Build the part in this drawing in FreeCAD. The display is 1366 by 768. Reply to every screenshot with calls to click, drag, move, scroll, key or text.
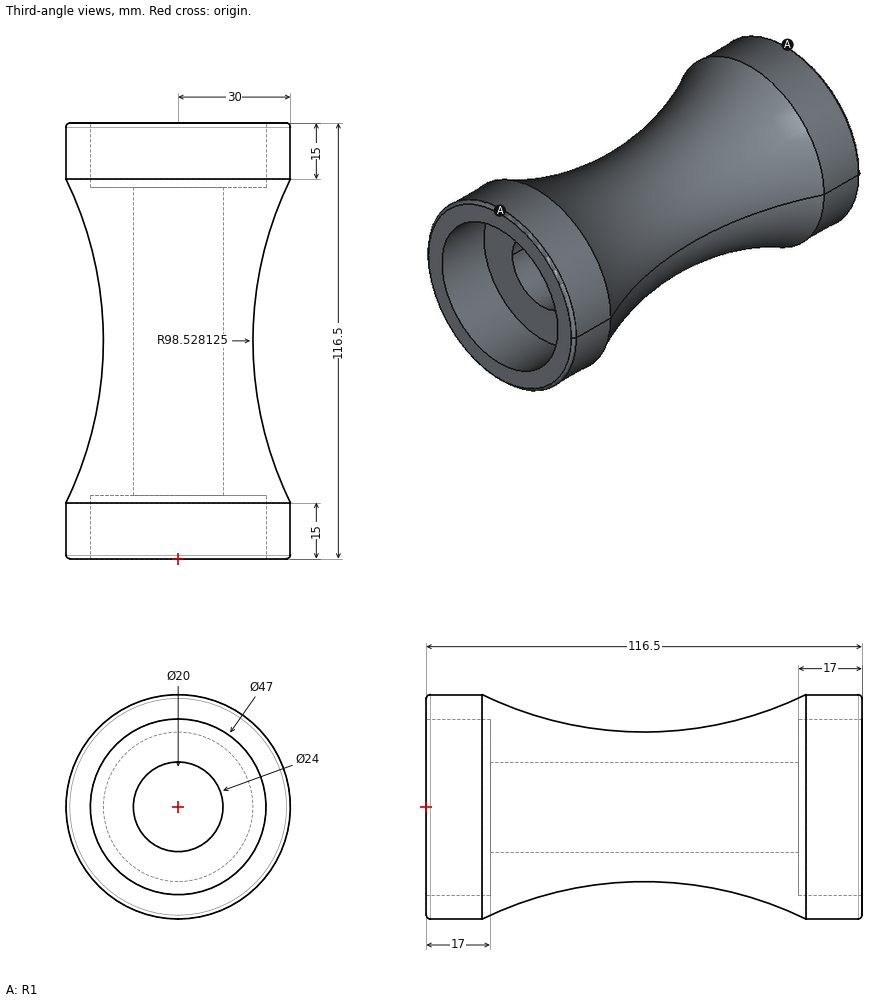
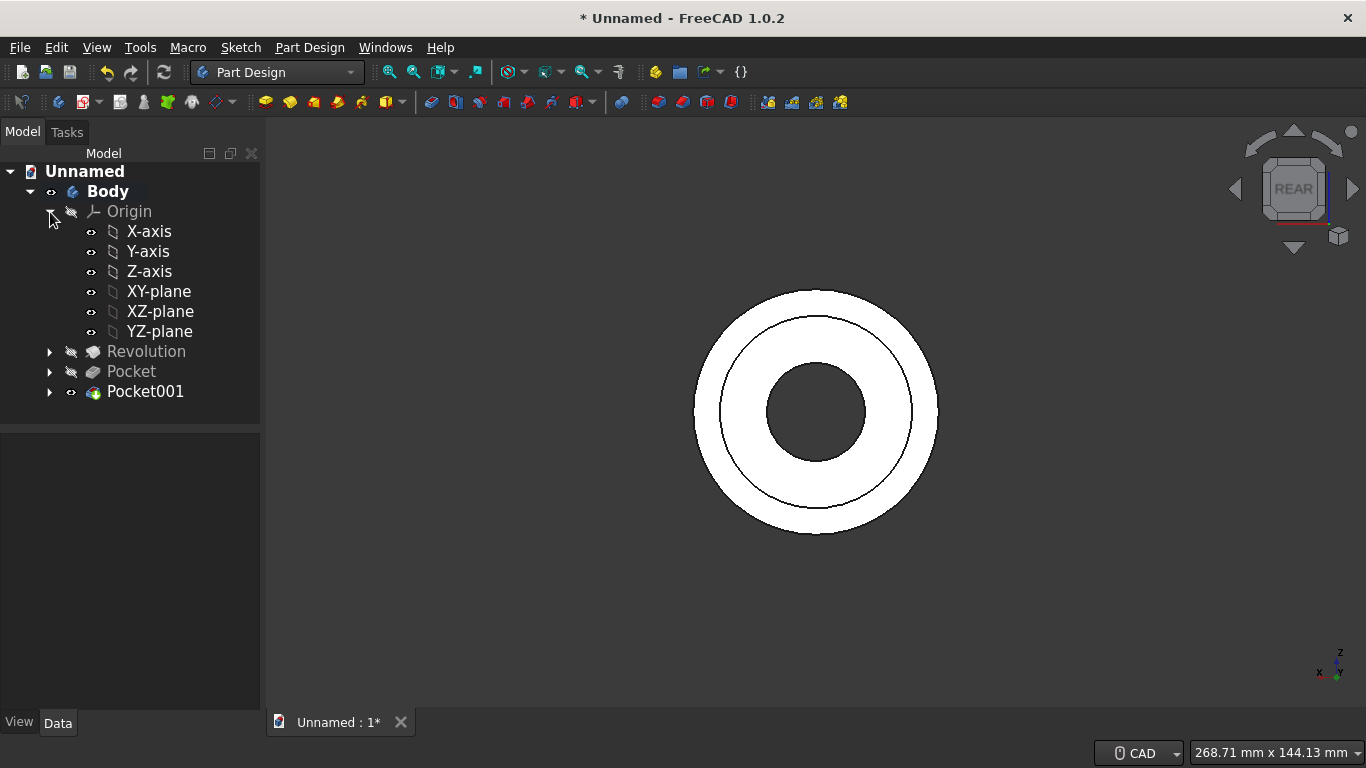
click(136, 312)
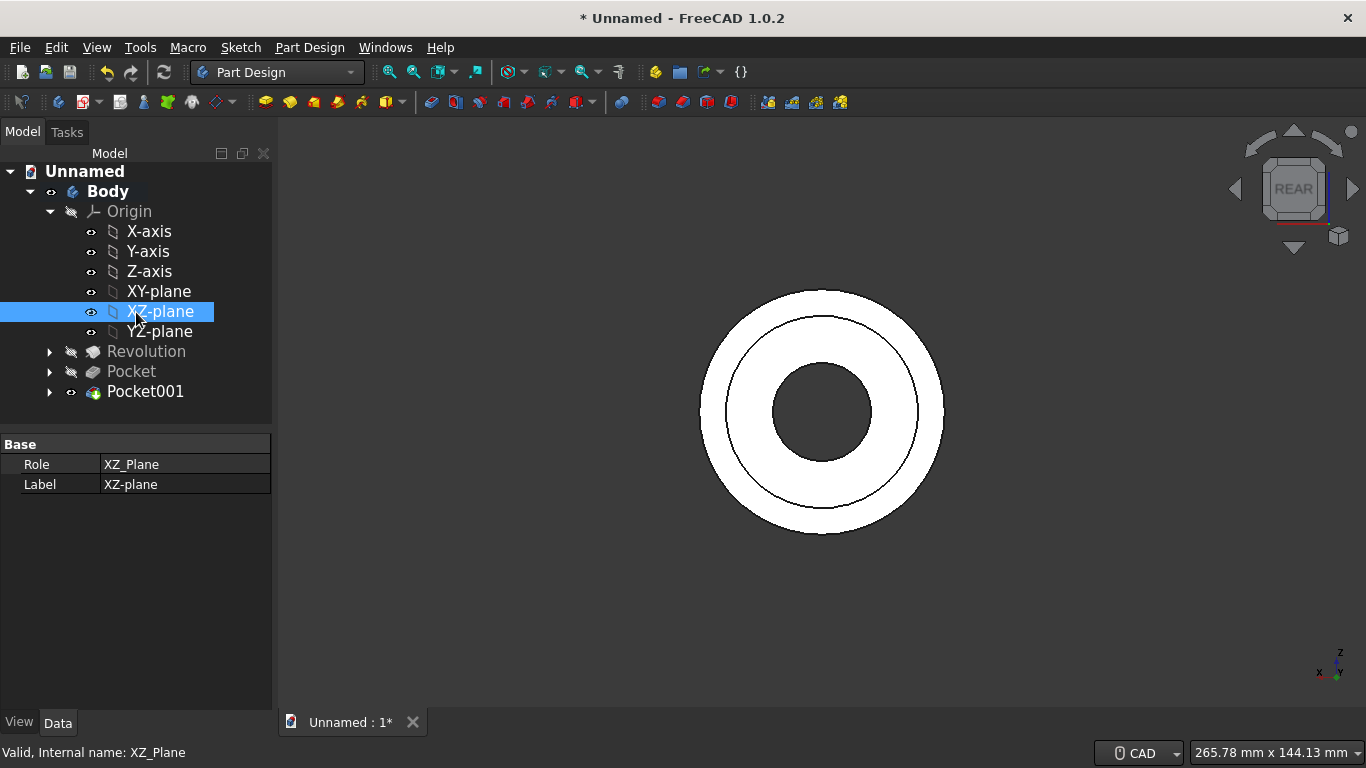
click(216, 102)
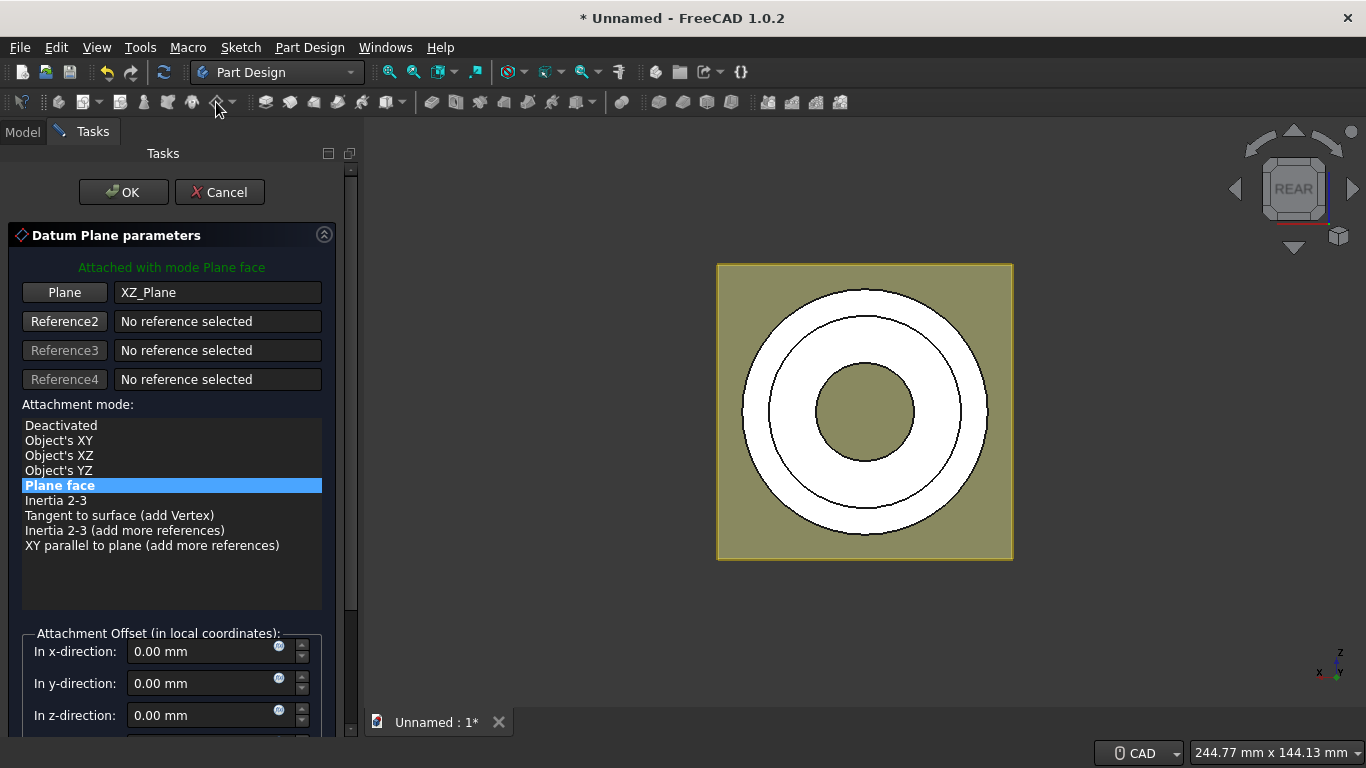
triple_click(210, 715)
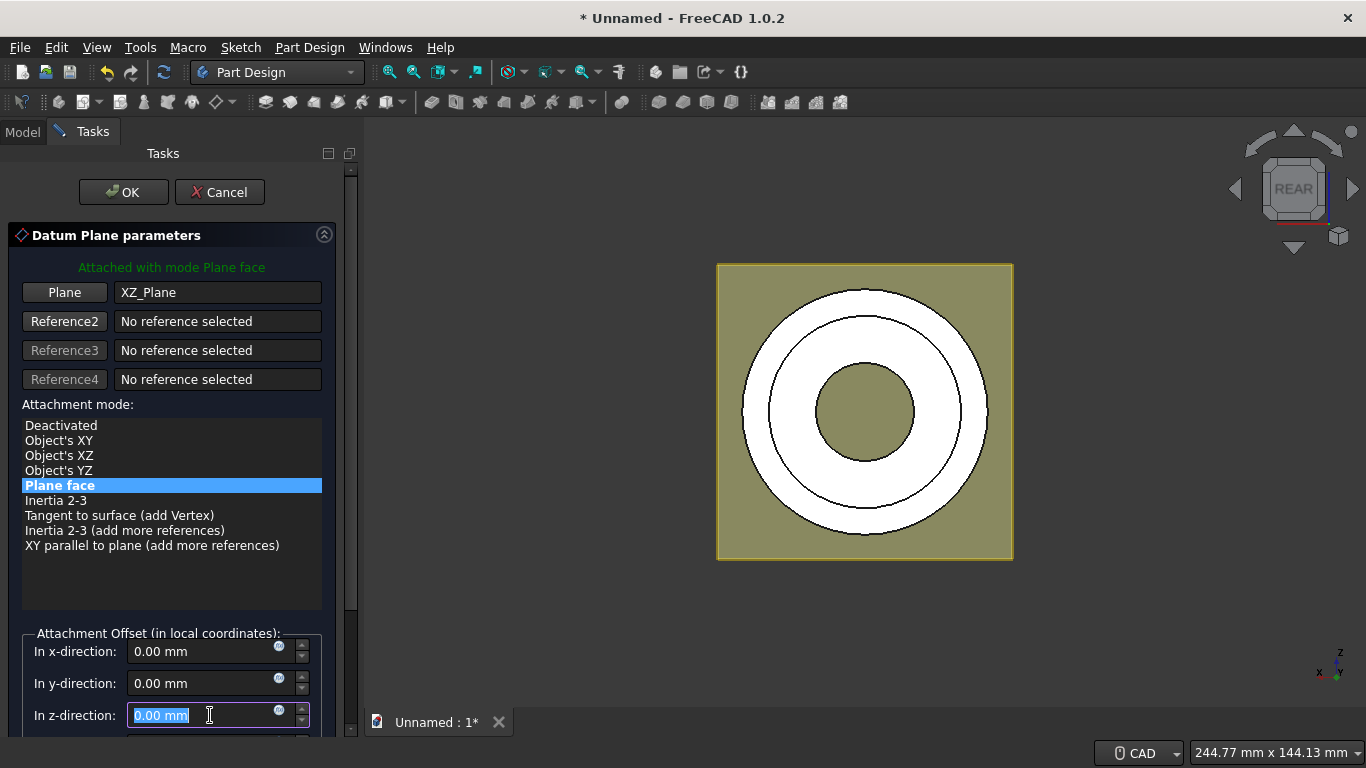
text(-17)
key(Tab)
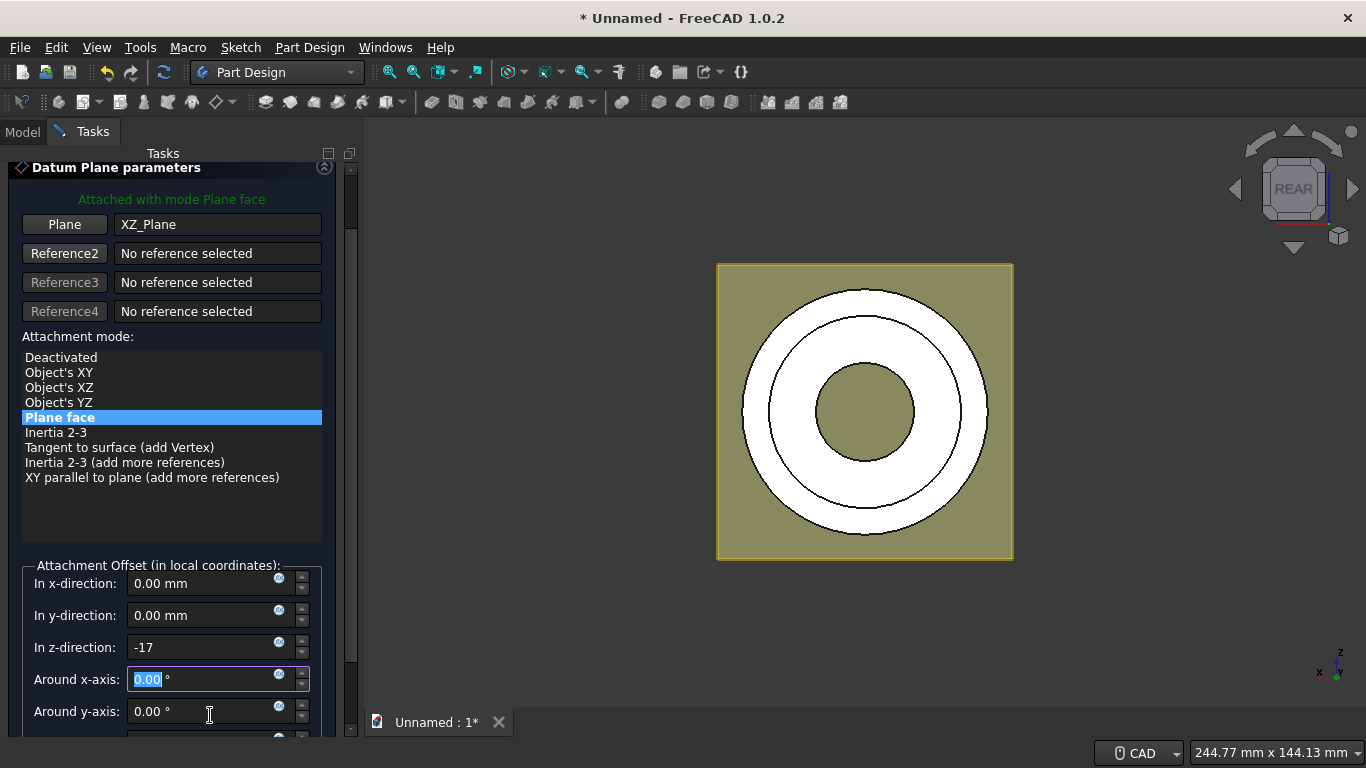
scroll(351, 450, up, 2)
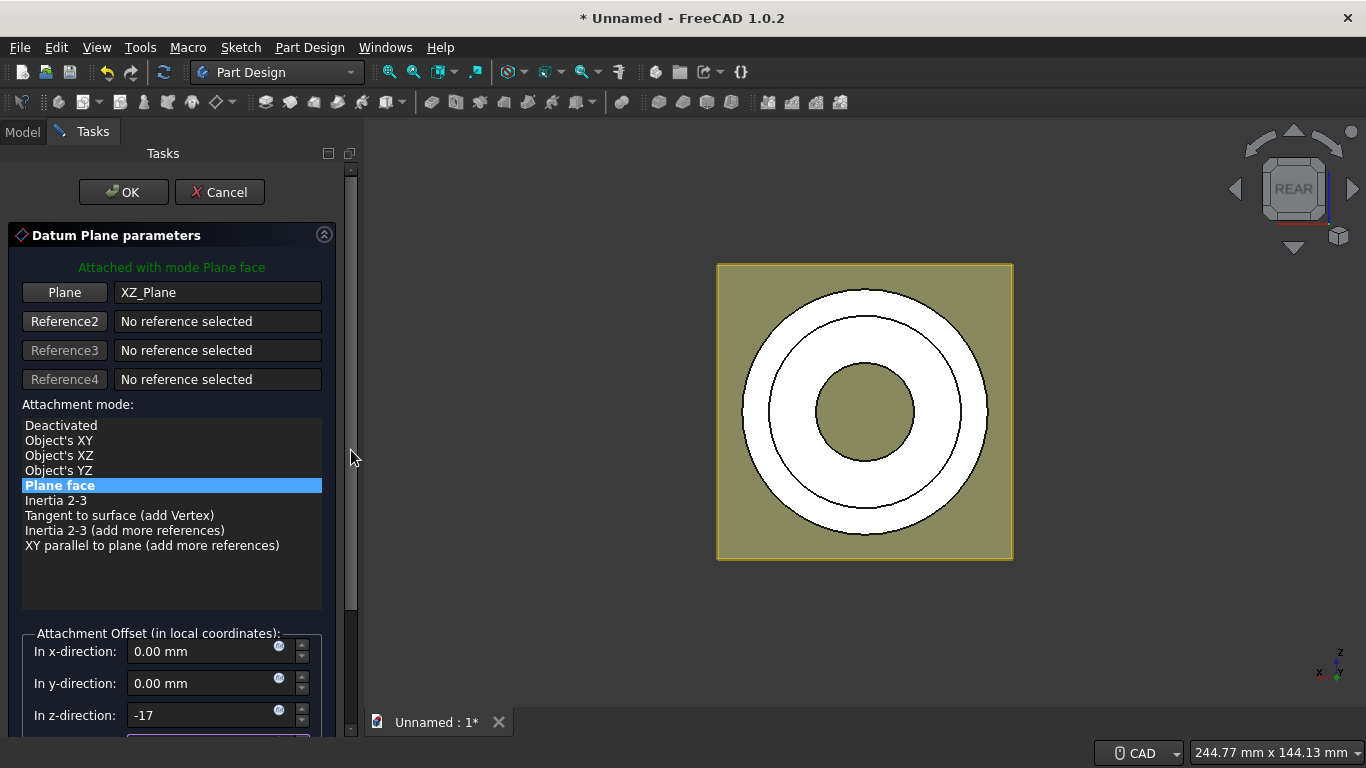
click(124, 192)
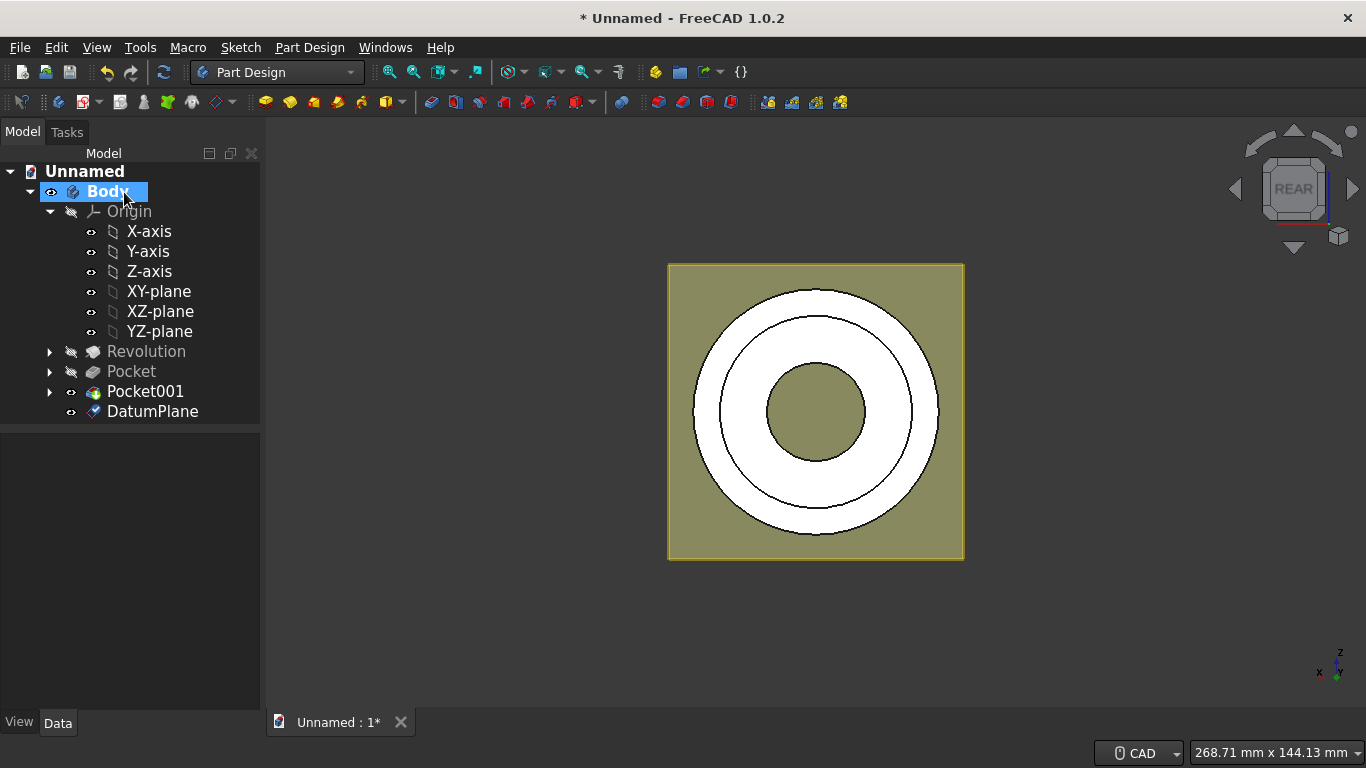
click(116, 412)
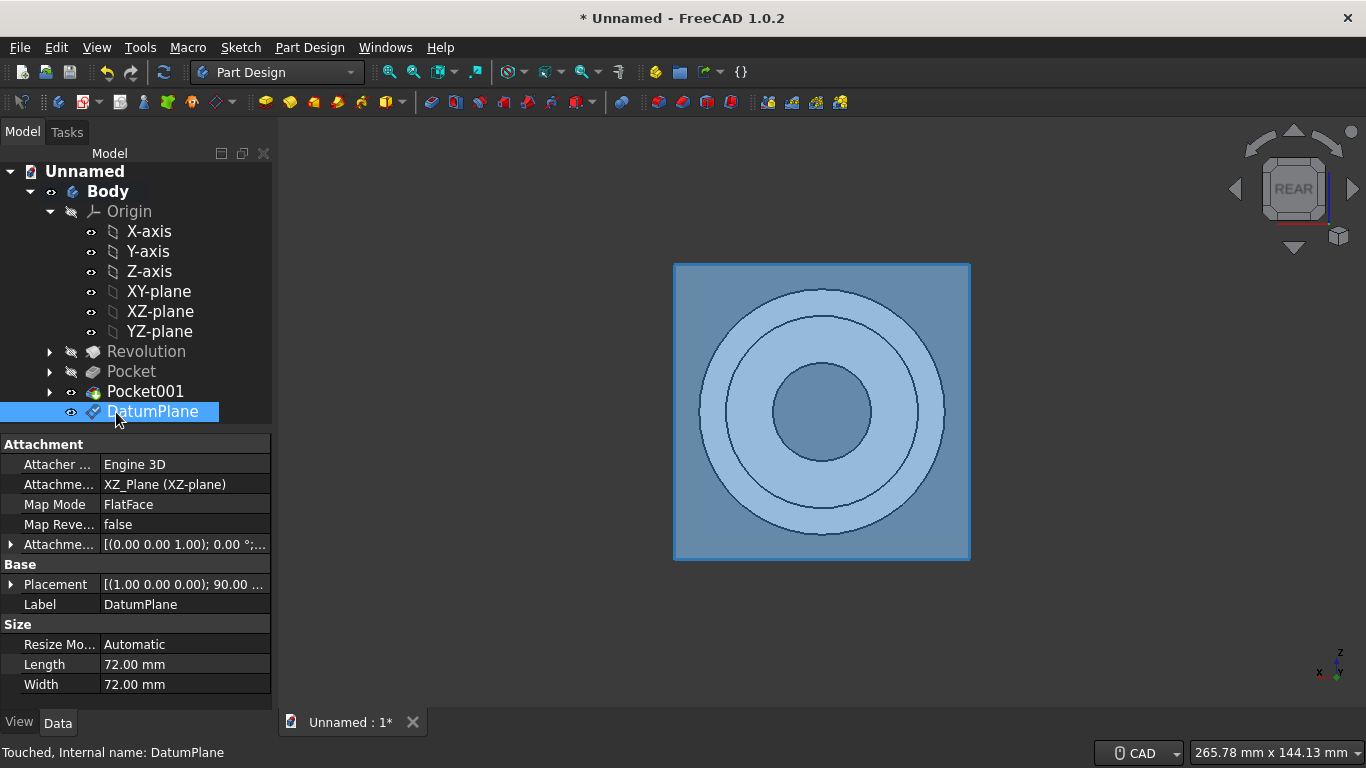
click(84, 102)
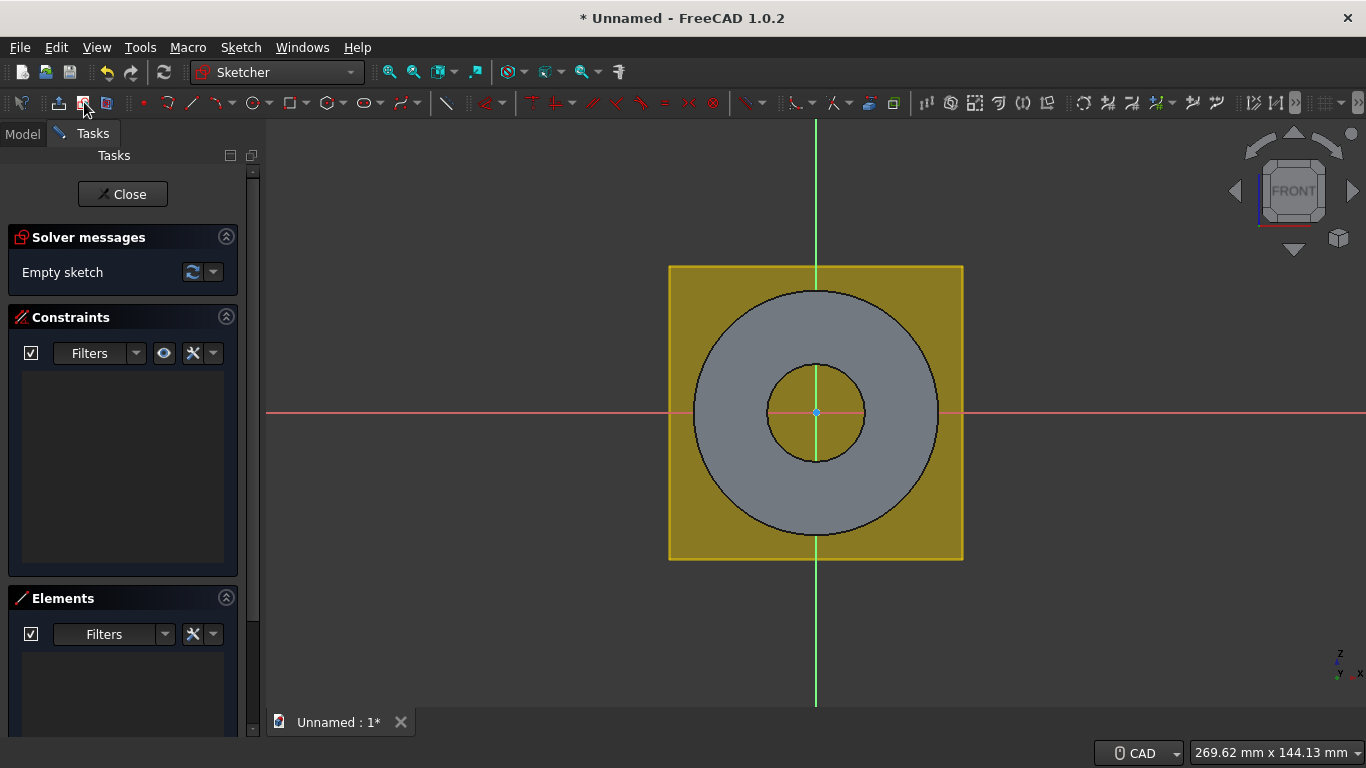
click(108, 104)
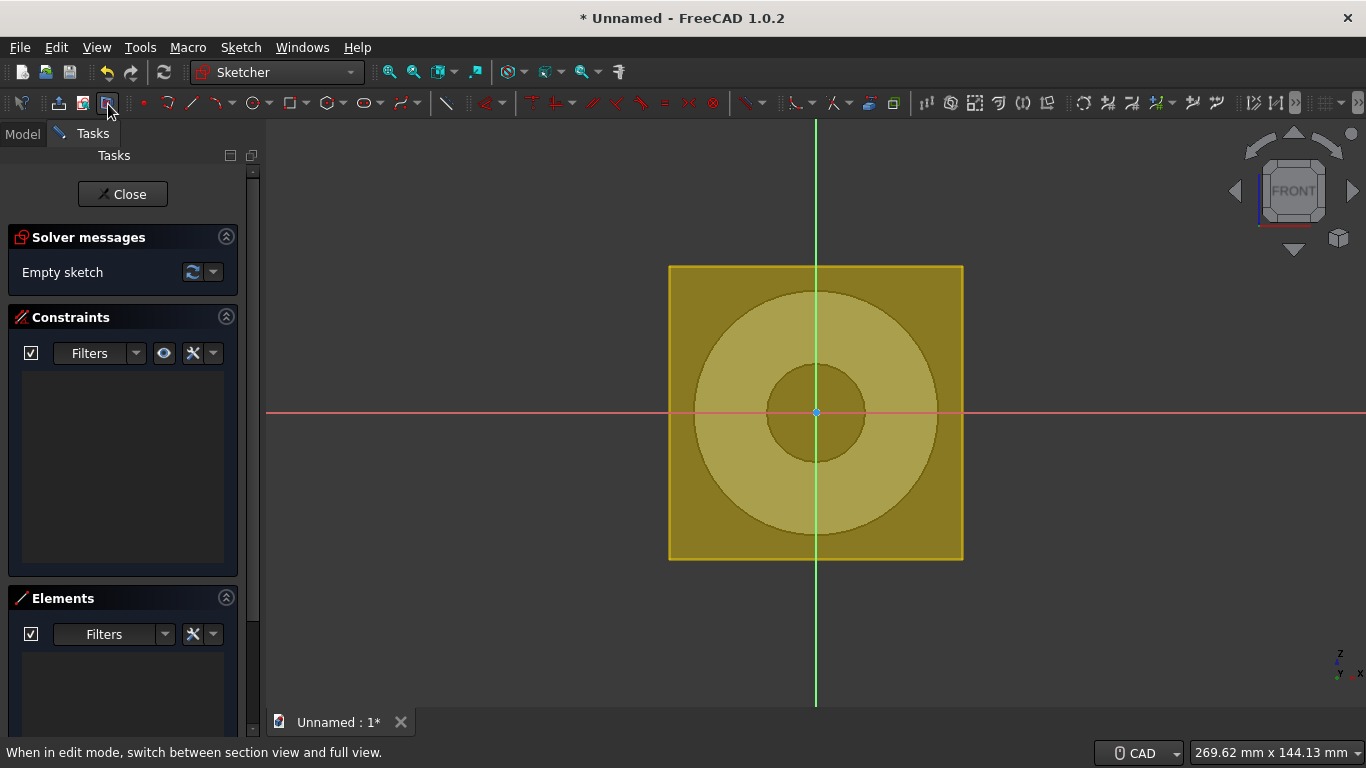
scroll(899, 413, up, 3)